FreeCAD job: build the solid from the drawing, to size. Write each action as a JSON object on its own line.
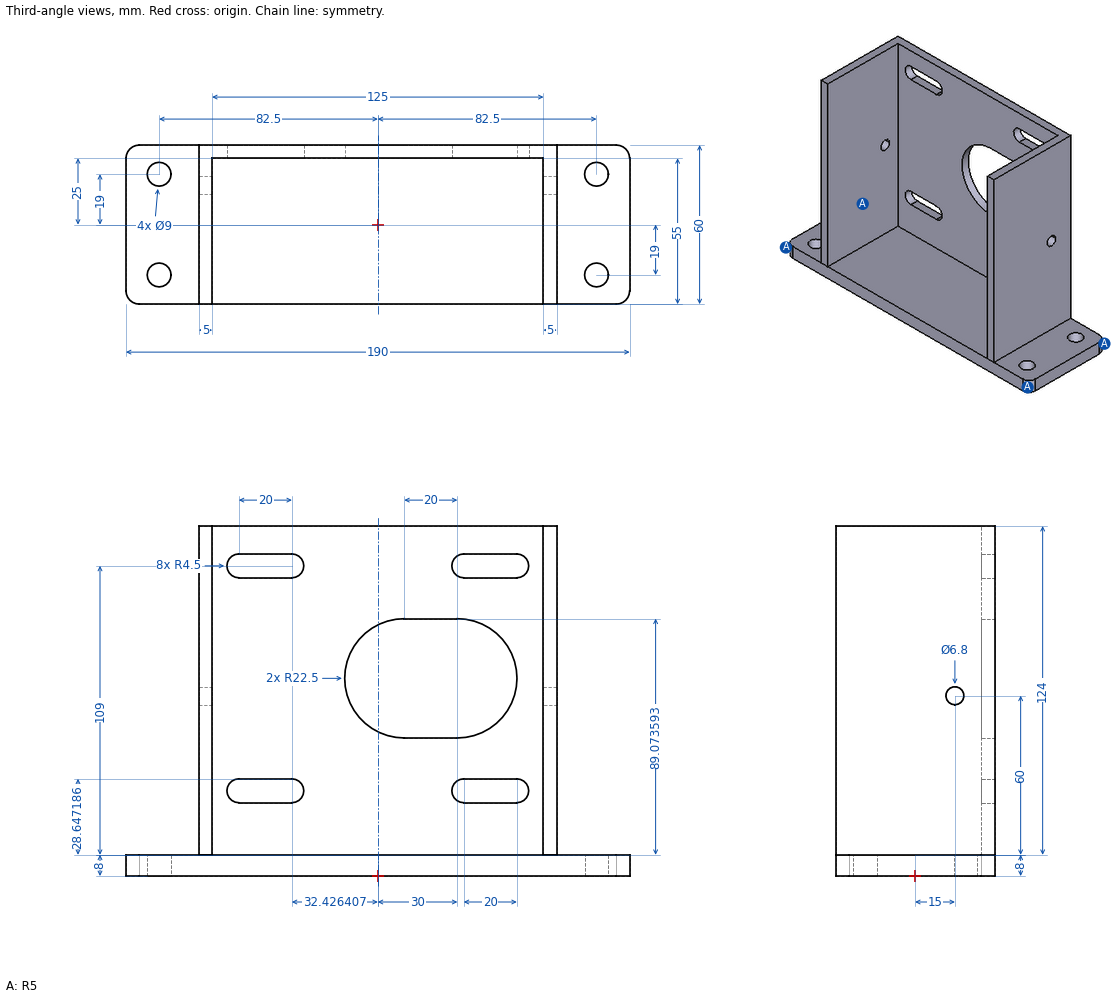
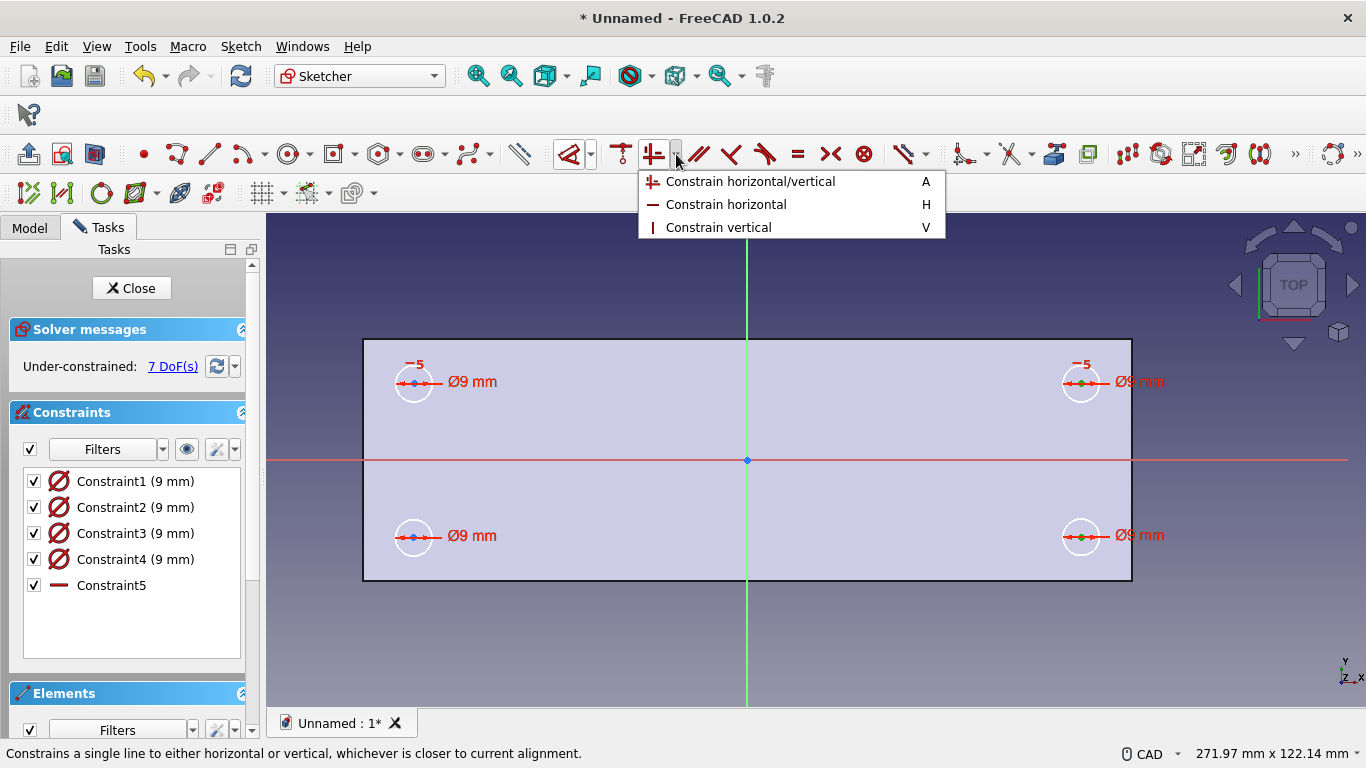
{"action": "left_click", "coordinate": [792, 228]}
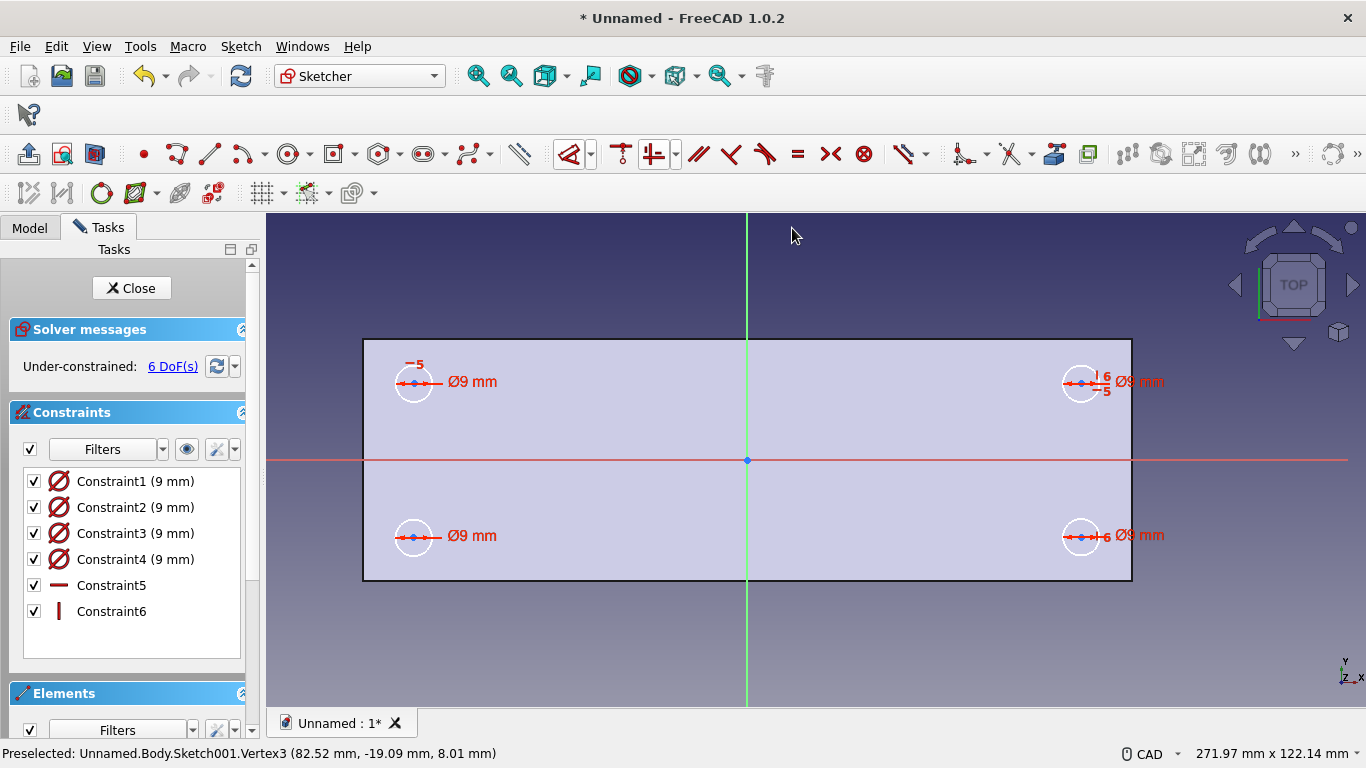
{"action": "left_click", "coordinate": [414, 384]}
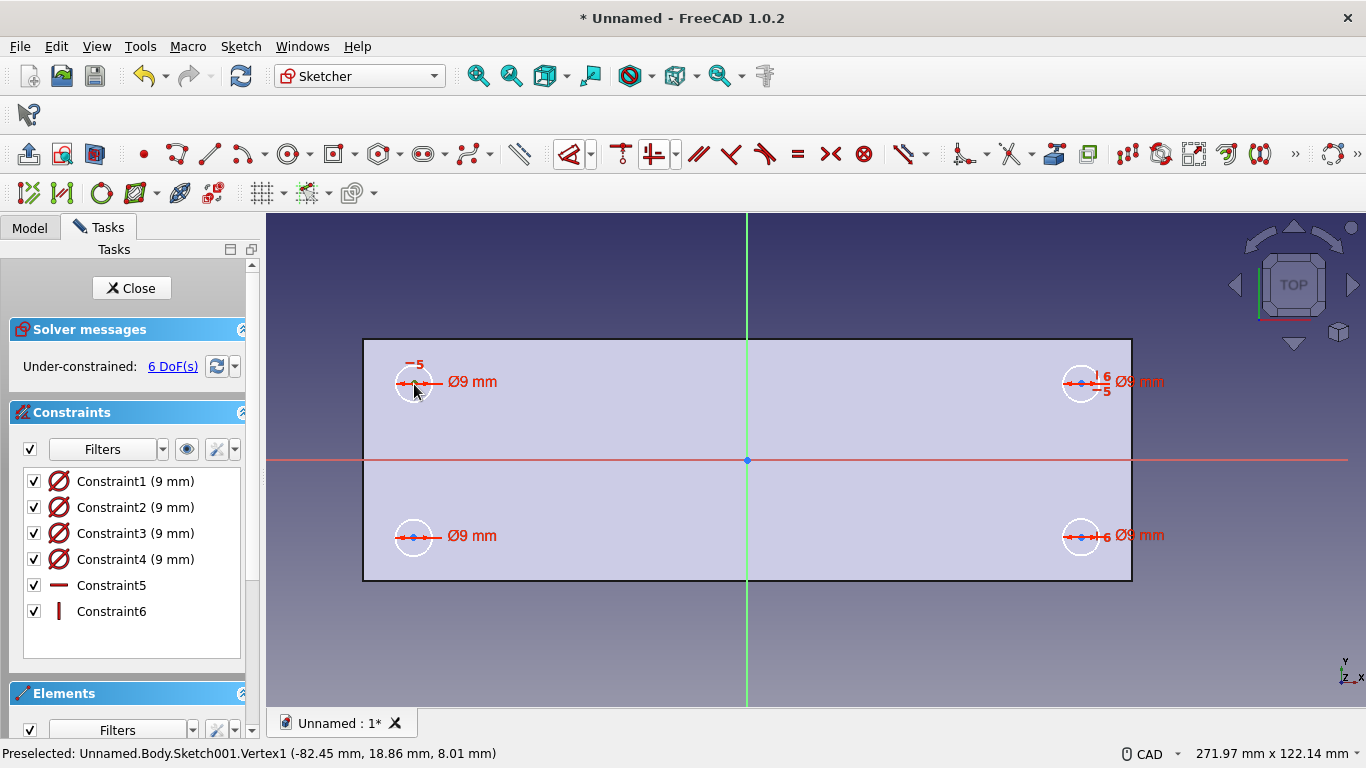
{"action": "left_click", "coordinate": [414, 538]}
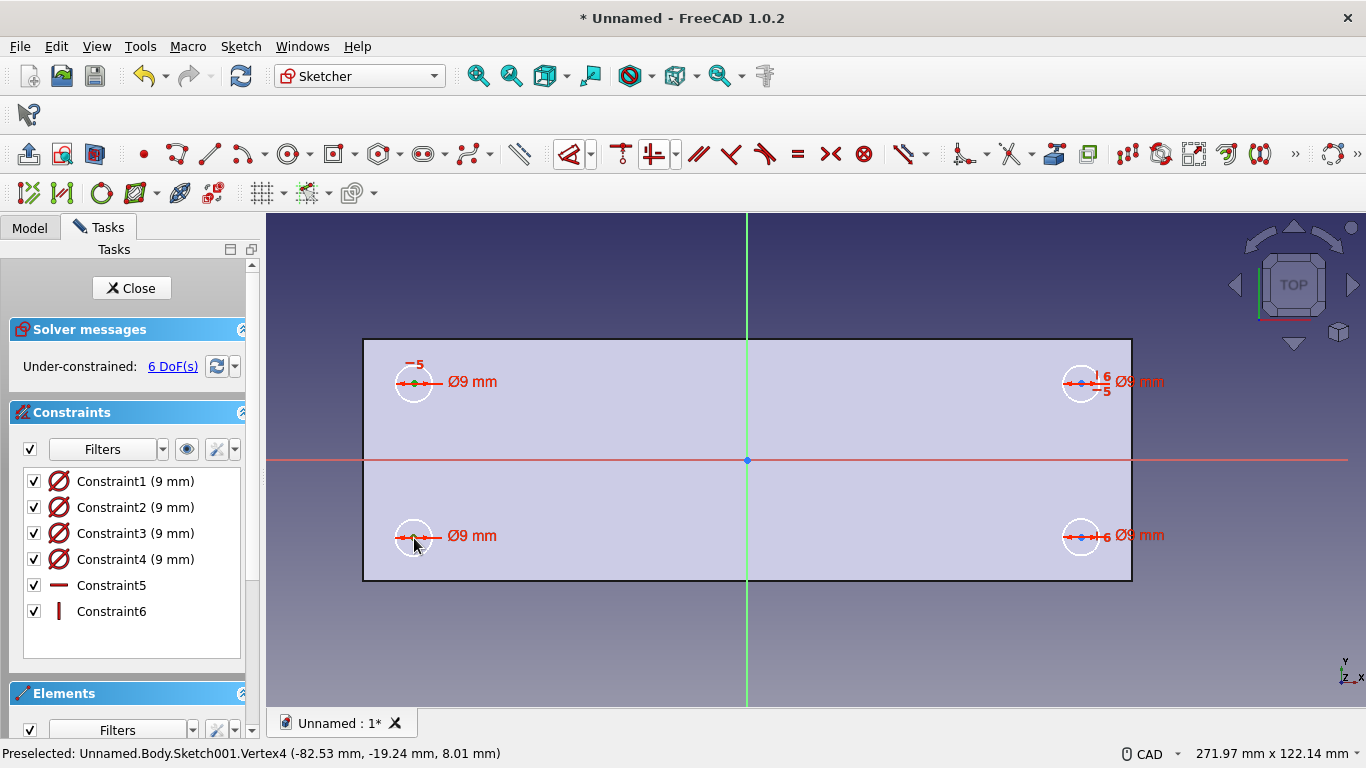
{"action": "left_click", "coordinate": [676, 154]}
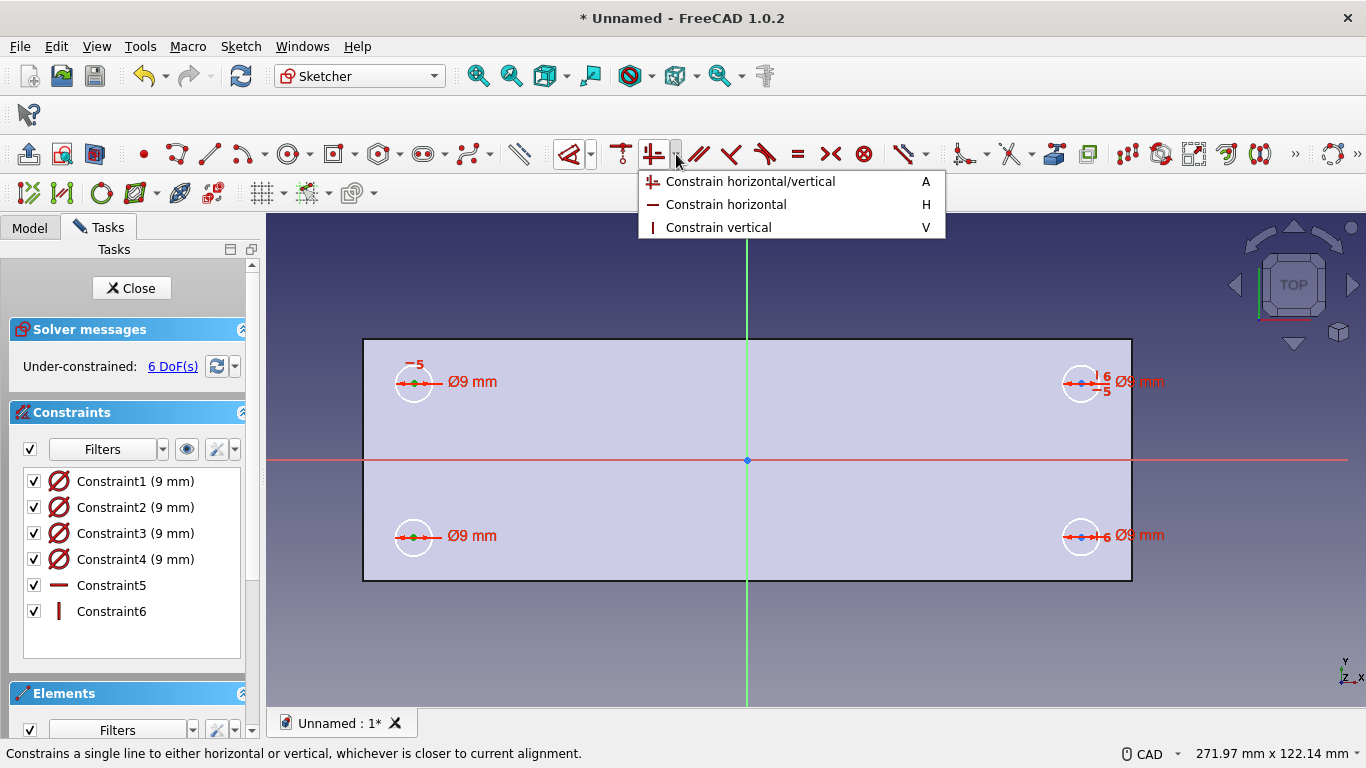
{"action": "left_click", "coordinate": [792, 228]}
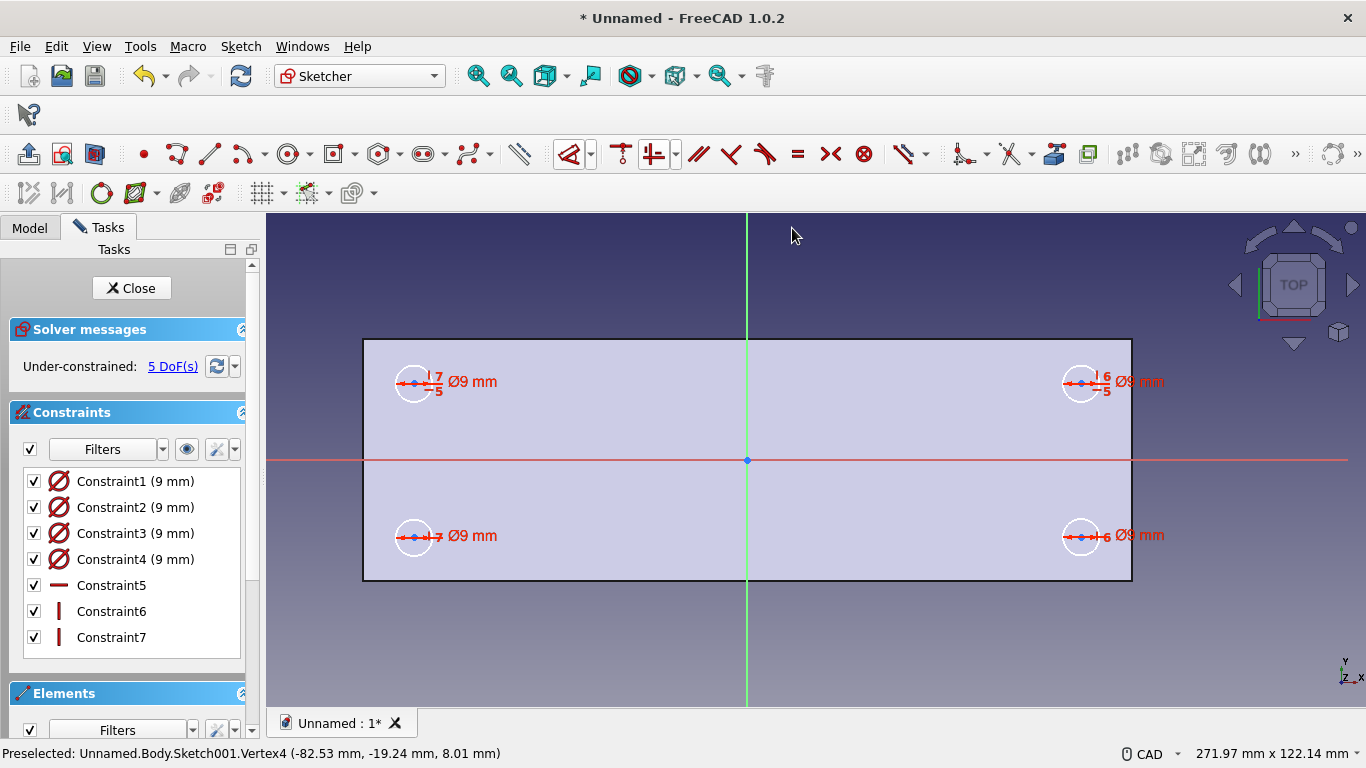
{"action": "left_click", "coordinate": [1081, 537]}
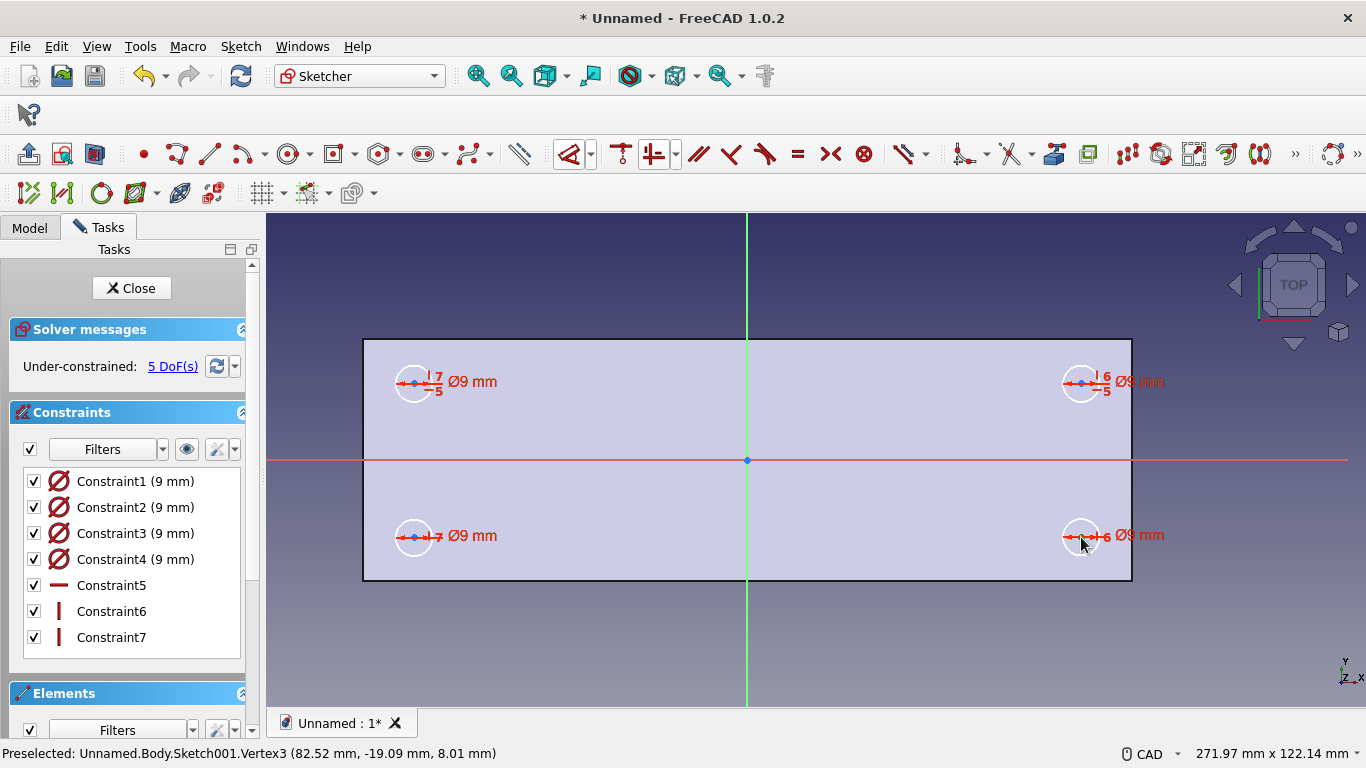
{"action": "left_click", "coordinate": [414, 538]}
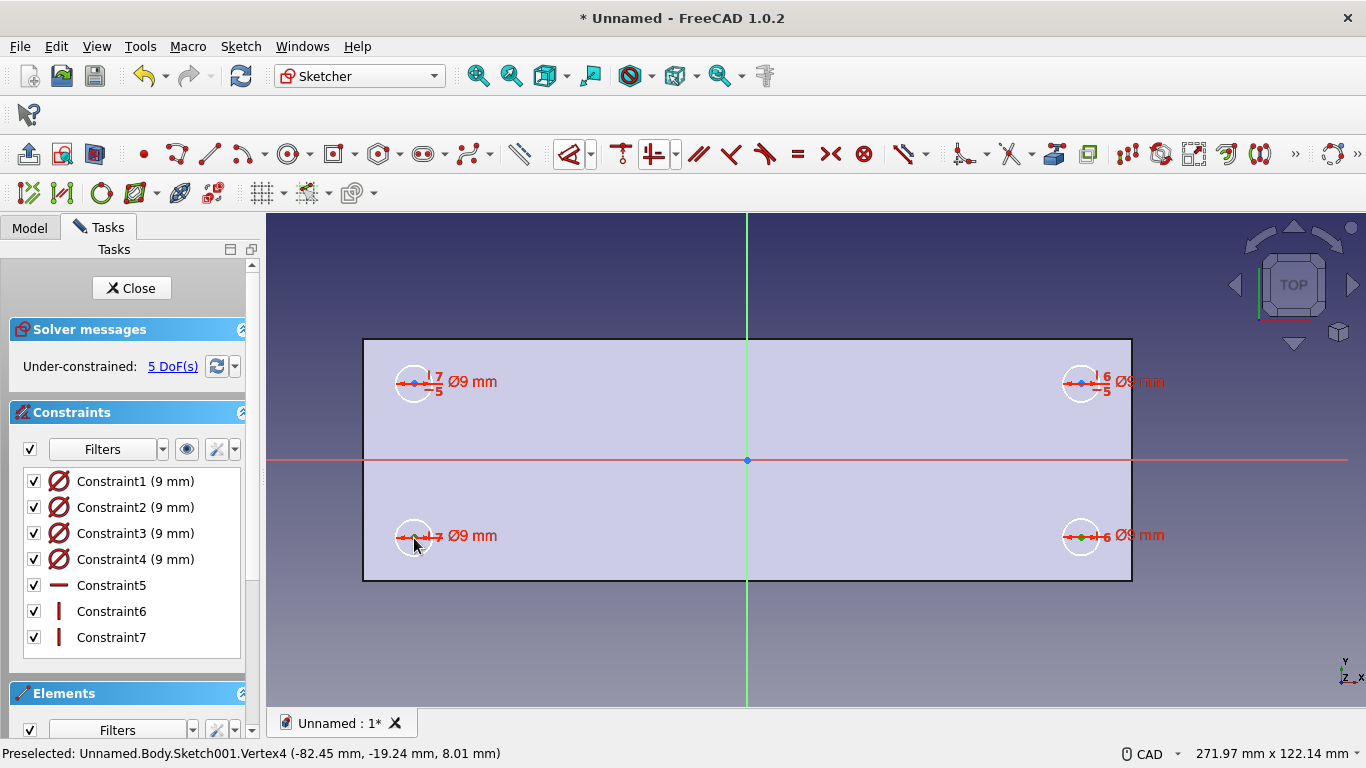
{"action": "left_click", "coordinate": [676, 154]}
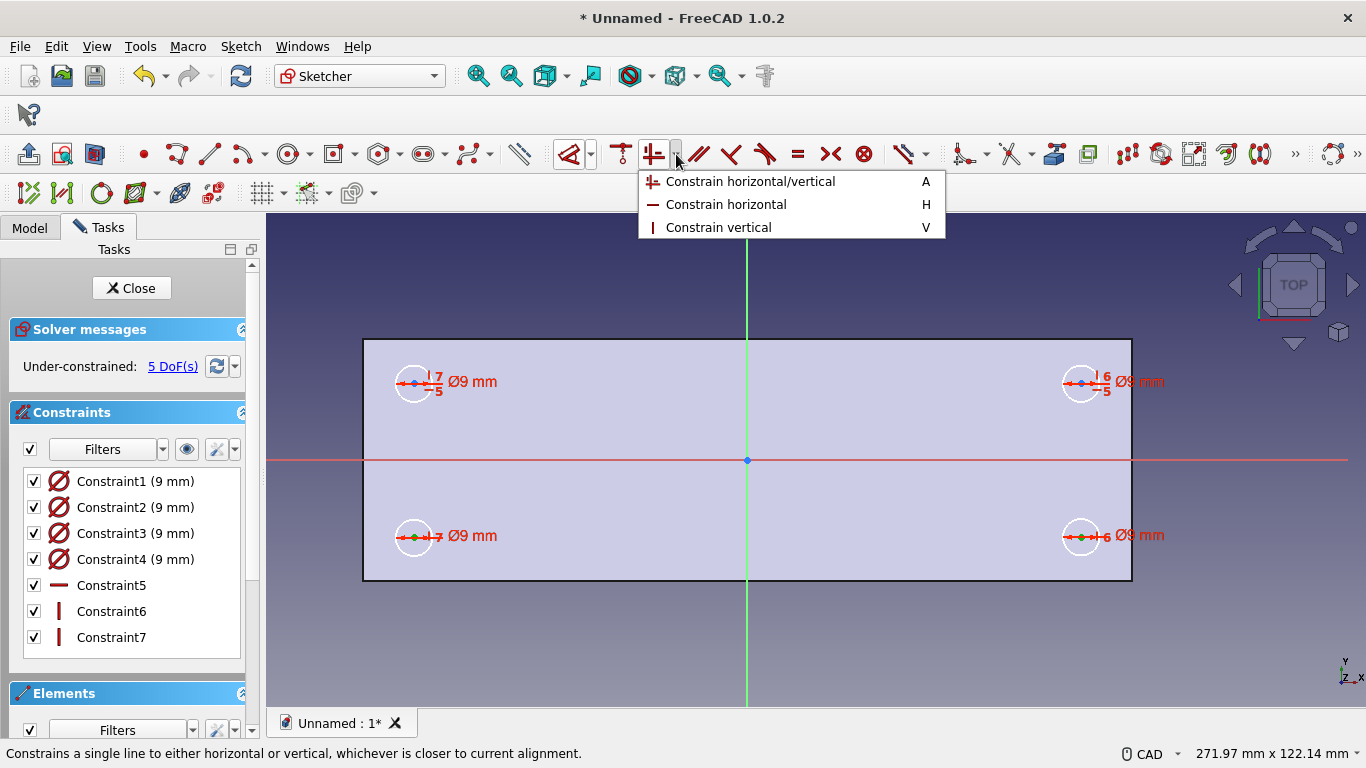
{"action": "left_click", "coordinate": [792, 204]}